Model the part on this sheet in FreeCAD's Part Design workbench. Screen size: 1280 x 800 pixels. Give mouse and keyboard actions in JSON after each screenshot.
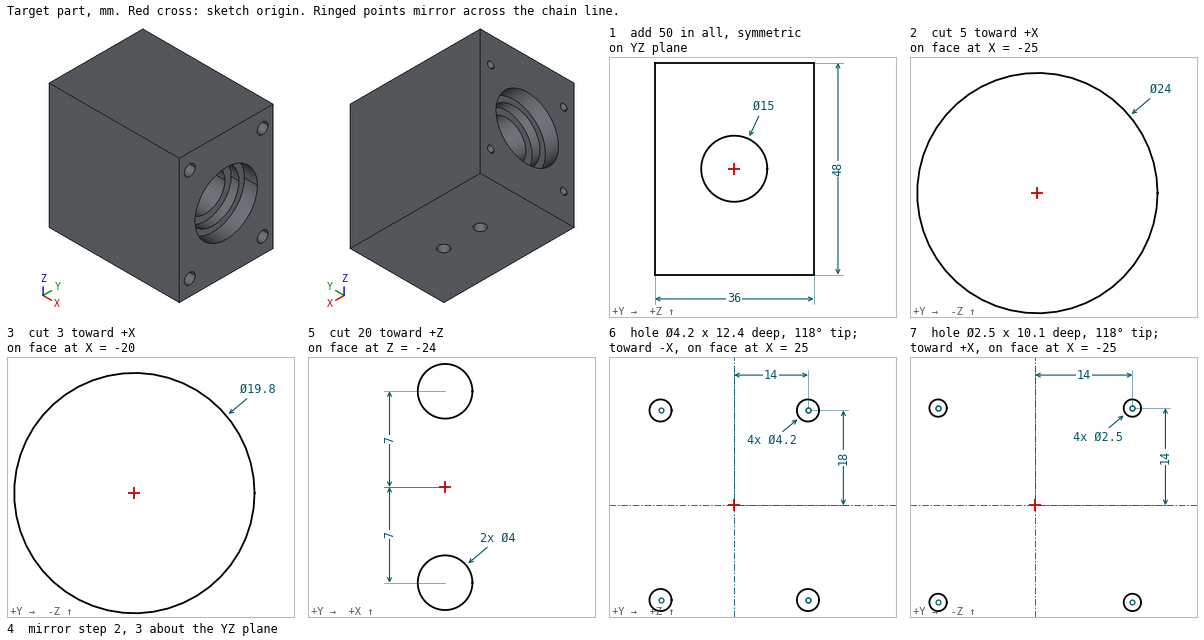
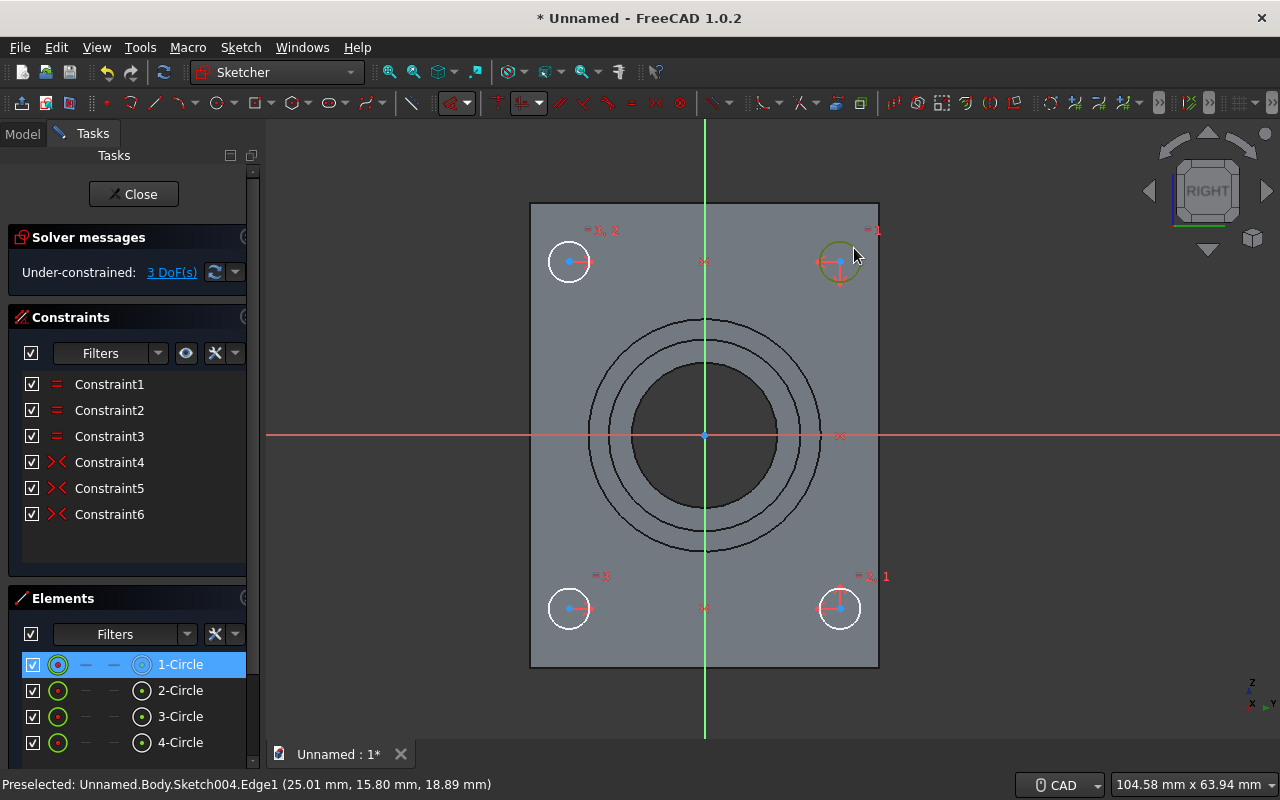
{"action": "key", "text": "k o"}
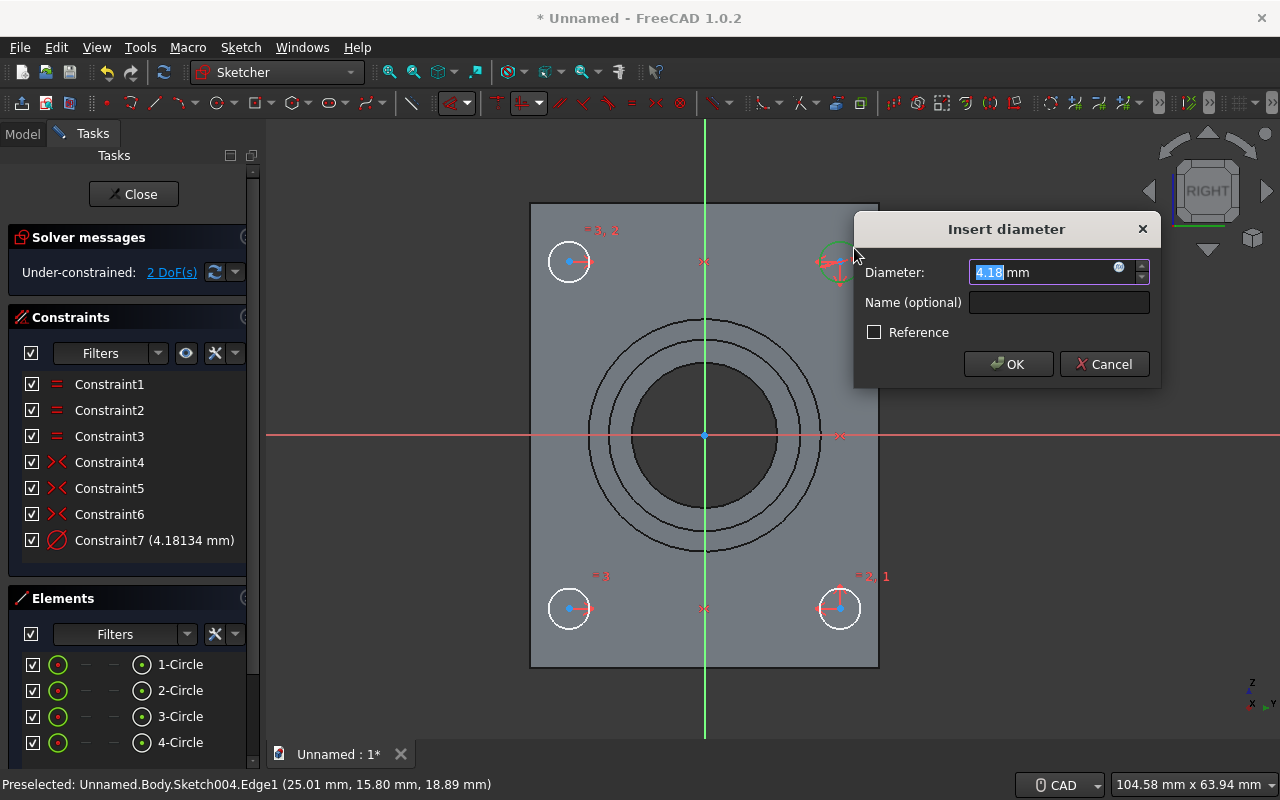
{"action": "type", "text": "4.2"}
{"action": "key", "text": "Return"}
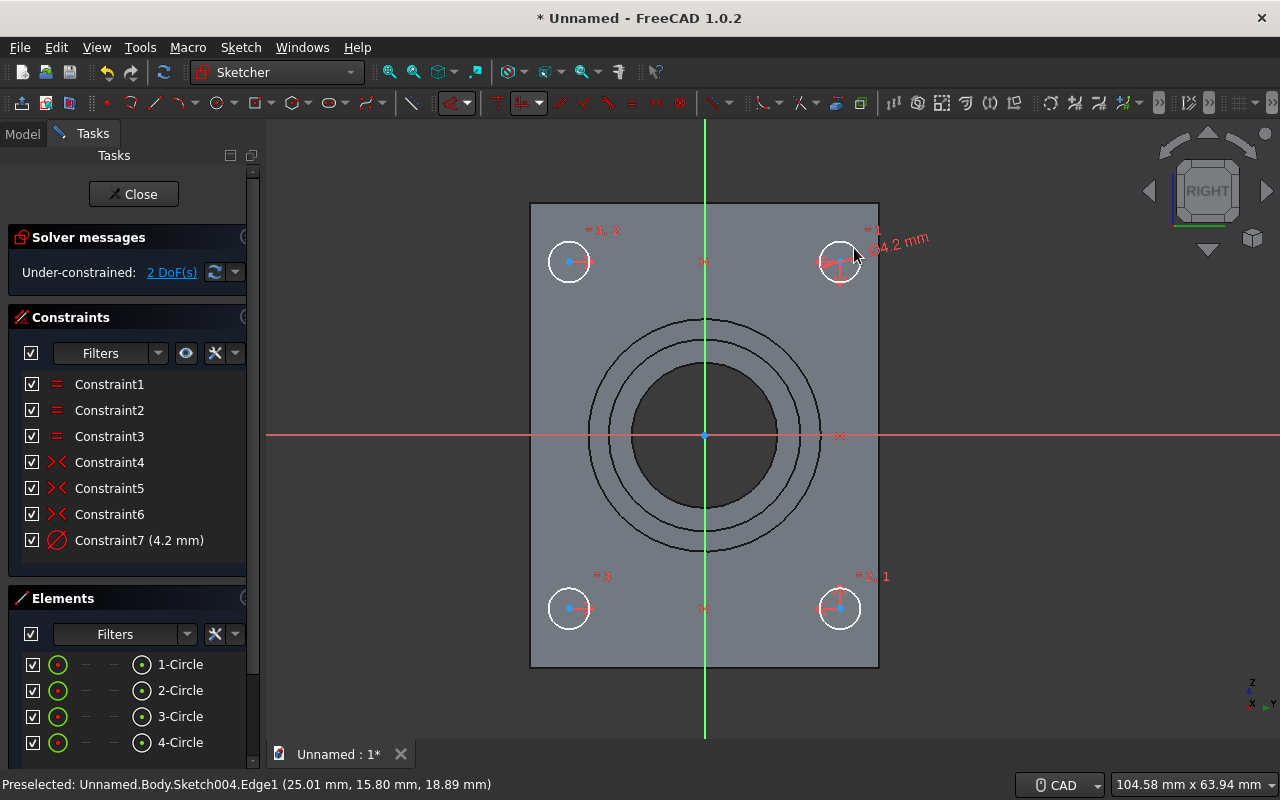
{"action": "left_click", "coordinate": [840, 262]}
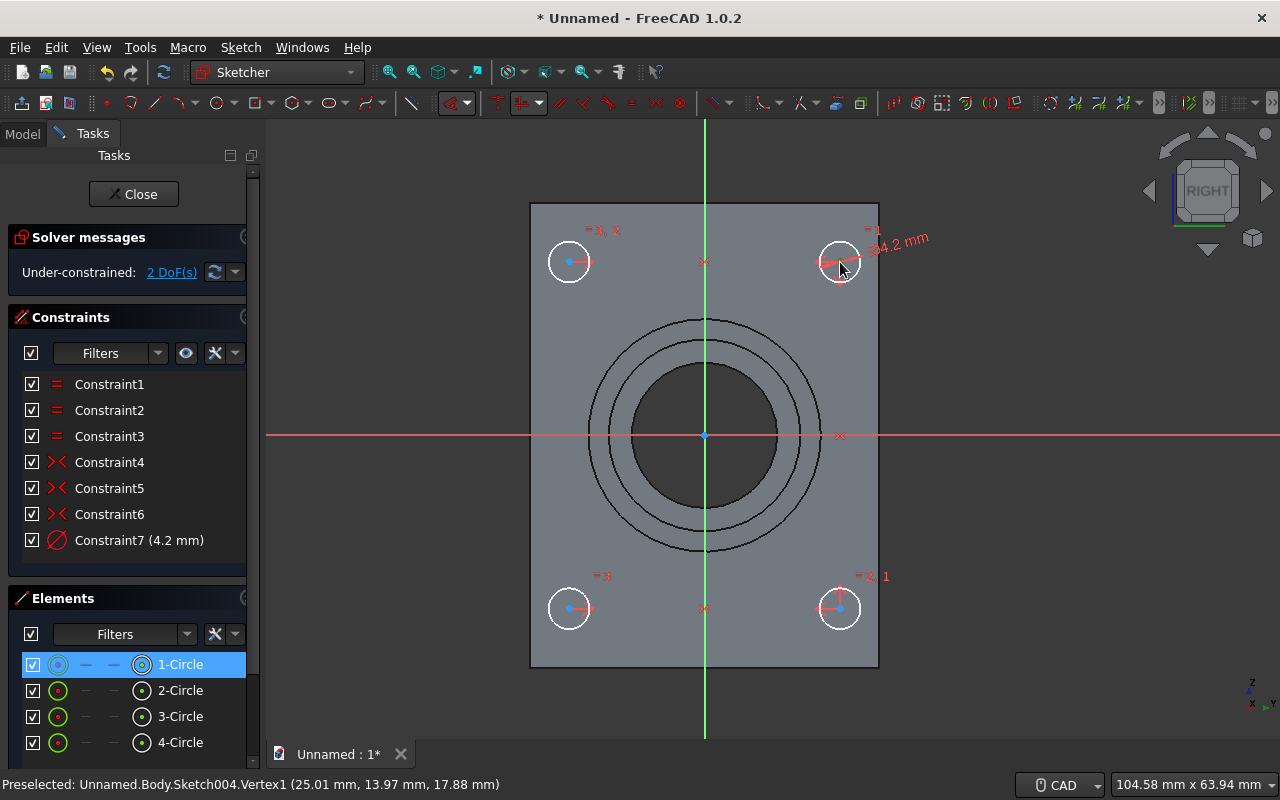
{"action": "key", "text": "l"}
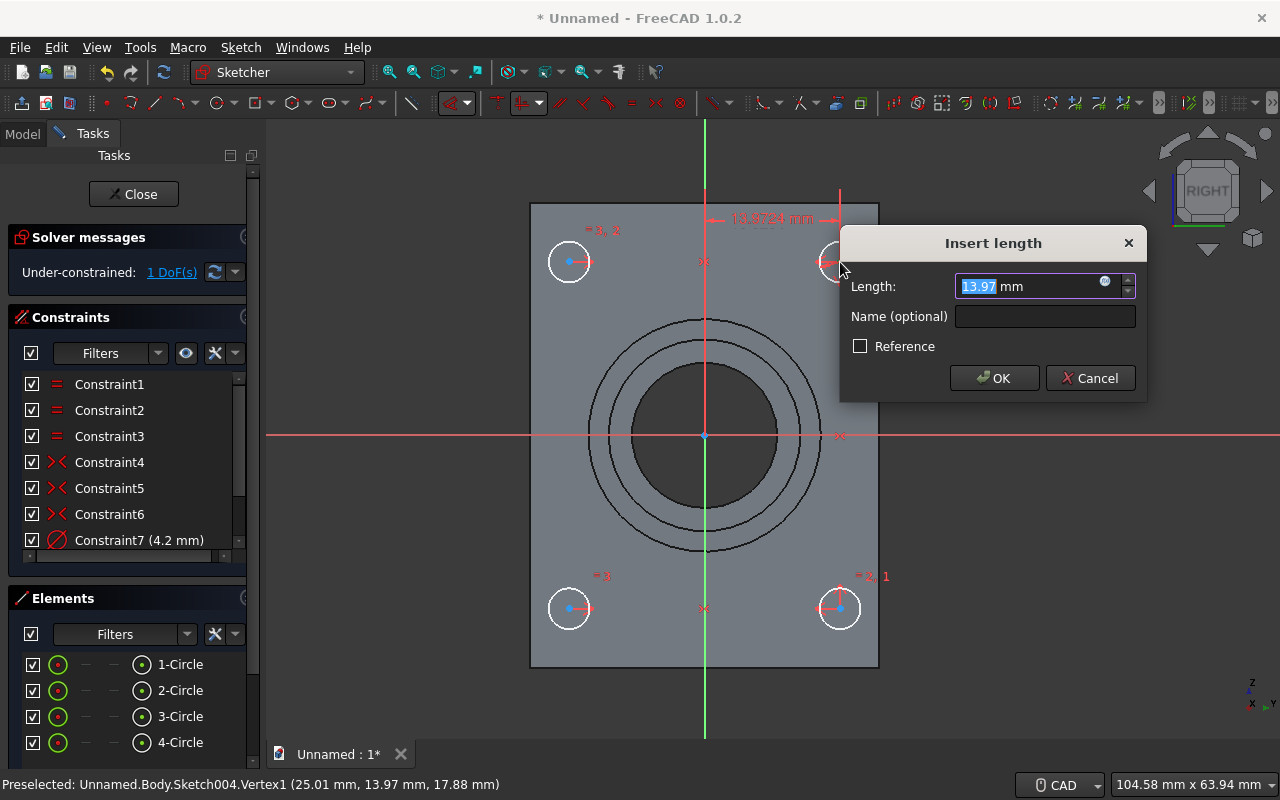
{"action": "type", "text": "14"}
{"action": "key", "text": "Return"}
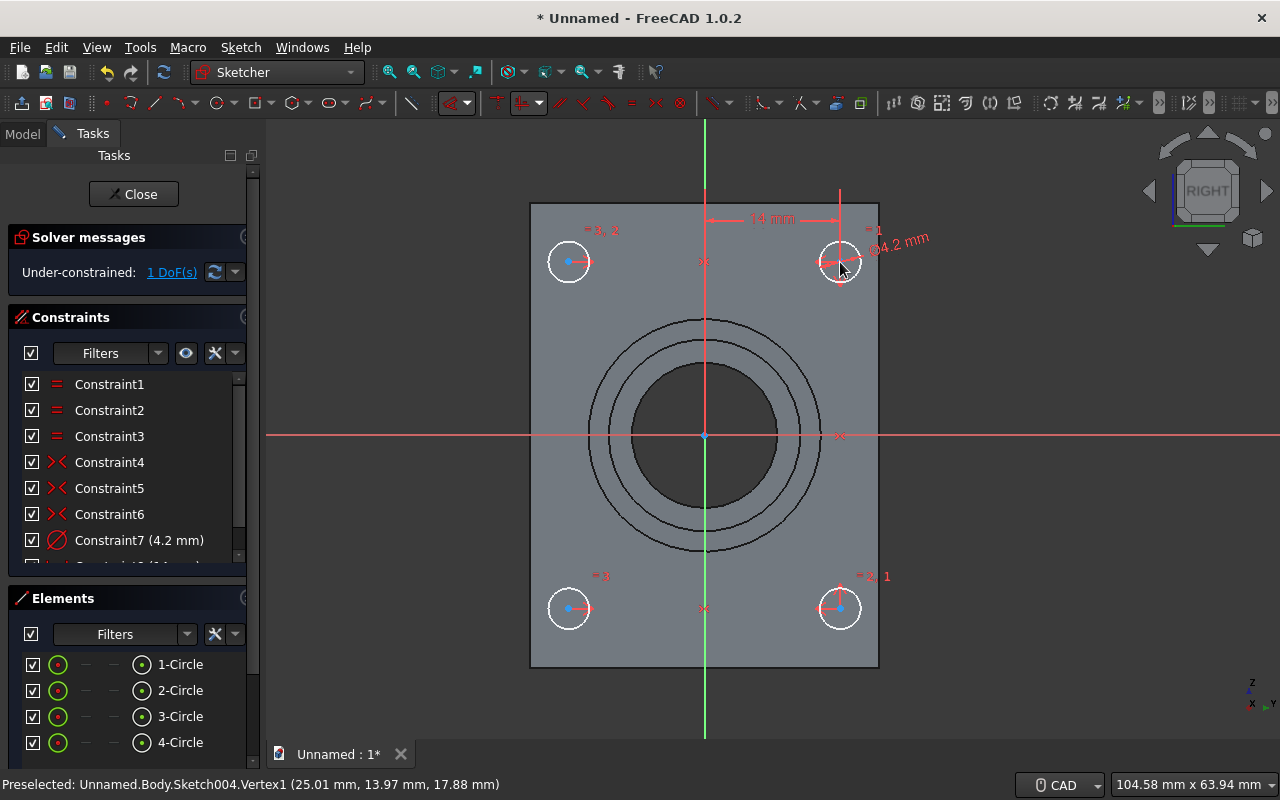
{"action": "left_click", "coordinate": [840, 262]}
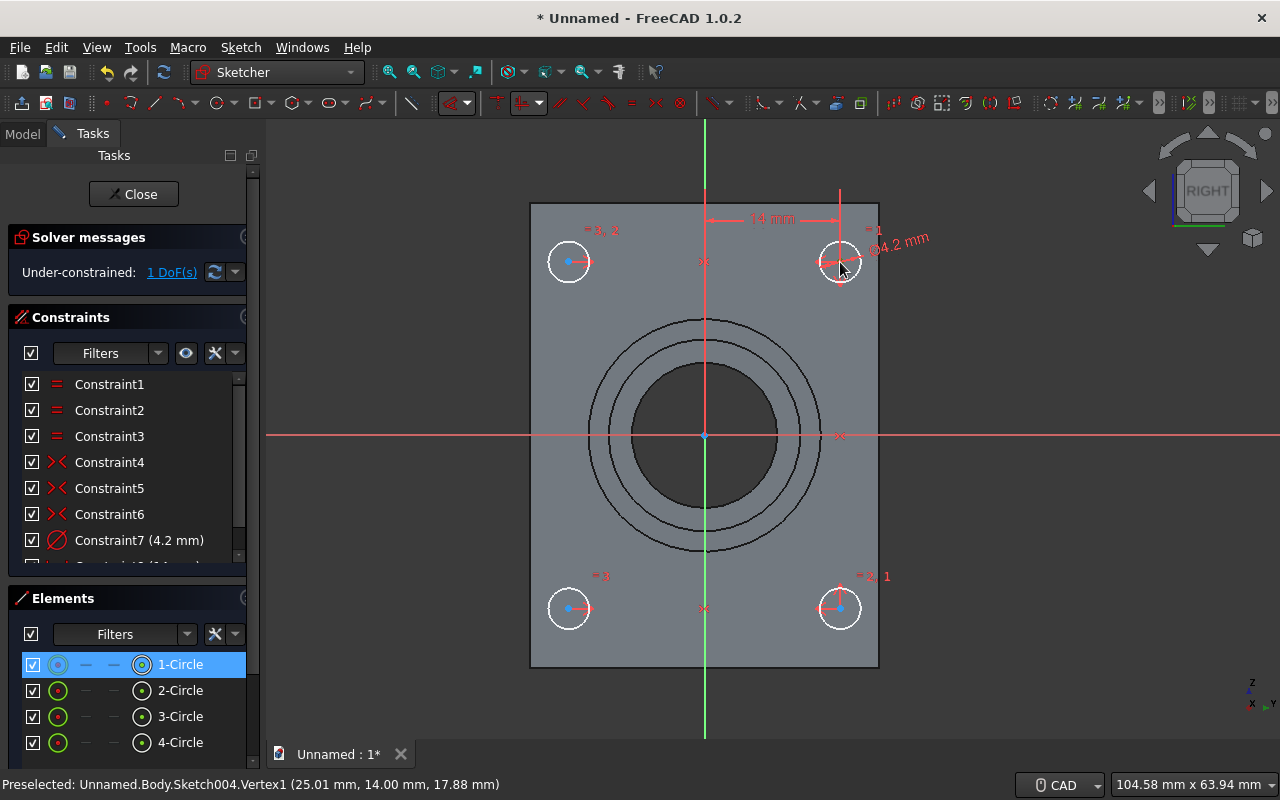
{"action": "left_click", "coordinate": [470, 104]}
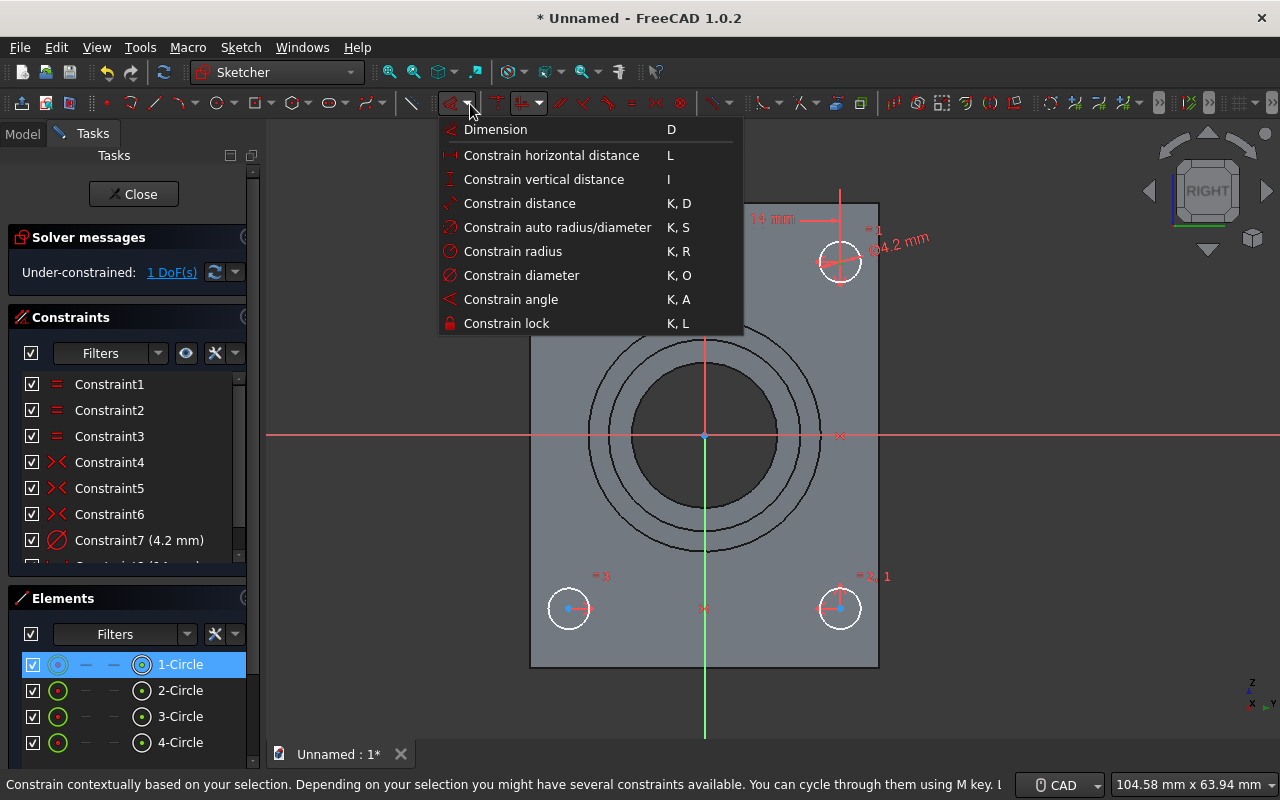
{"action": "left_click", "coordinate": [591, 179]}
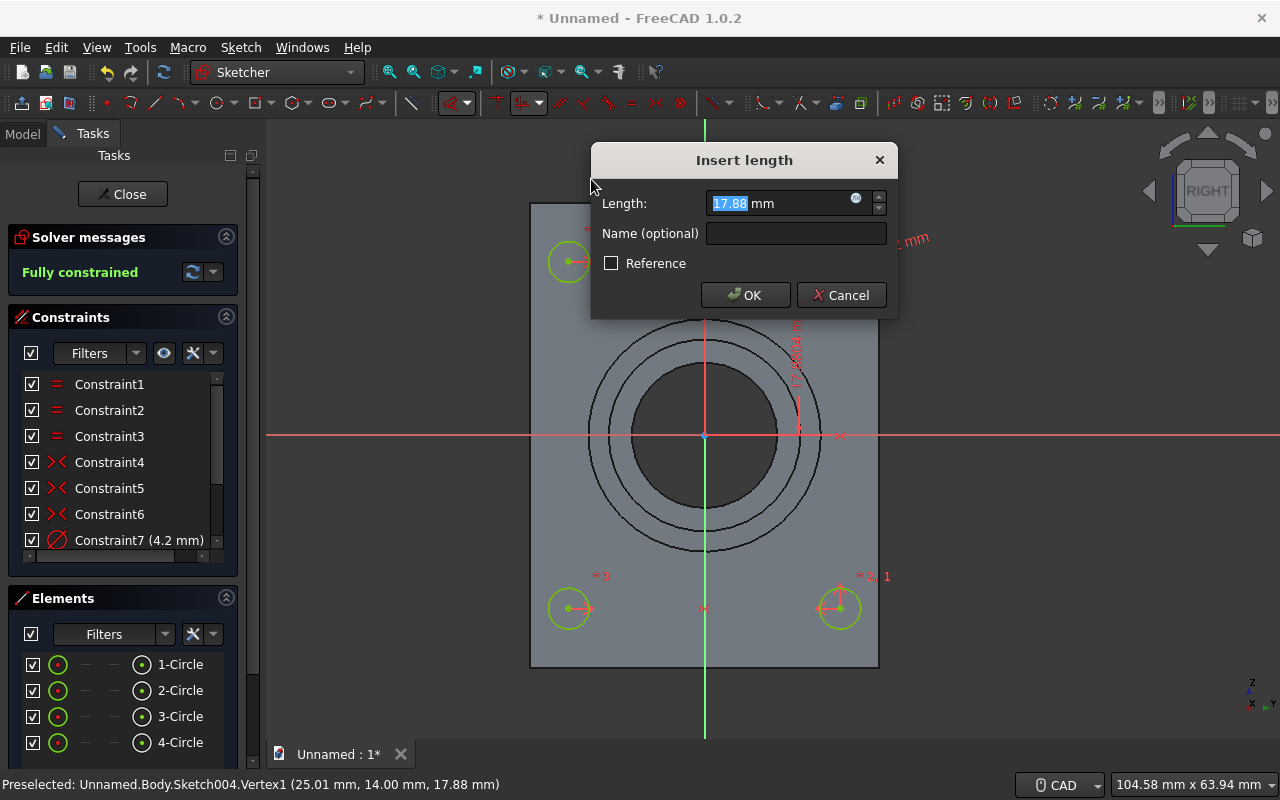
{"action": "type", "text": "18"}
{"action": "key", "text": "Return"}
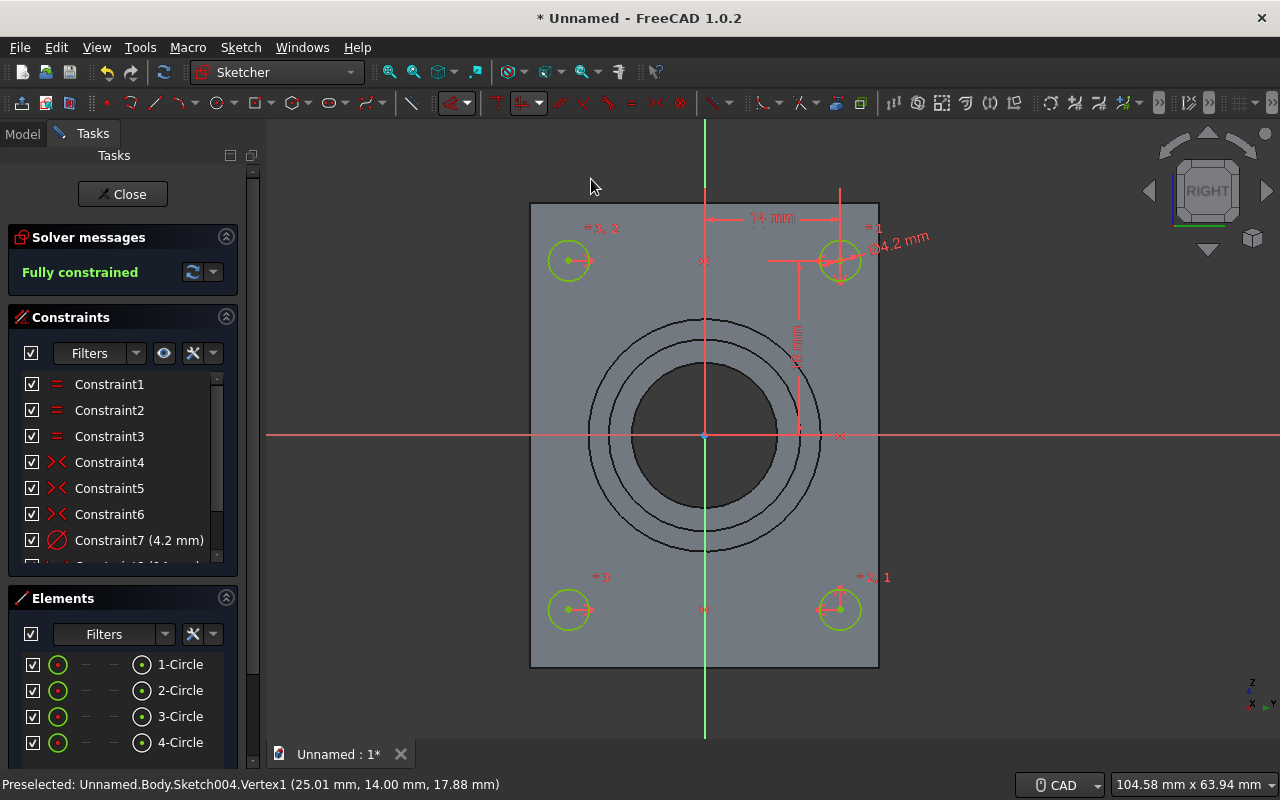
{"action": "left_click", "coordinate": [123, 194]}